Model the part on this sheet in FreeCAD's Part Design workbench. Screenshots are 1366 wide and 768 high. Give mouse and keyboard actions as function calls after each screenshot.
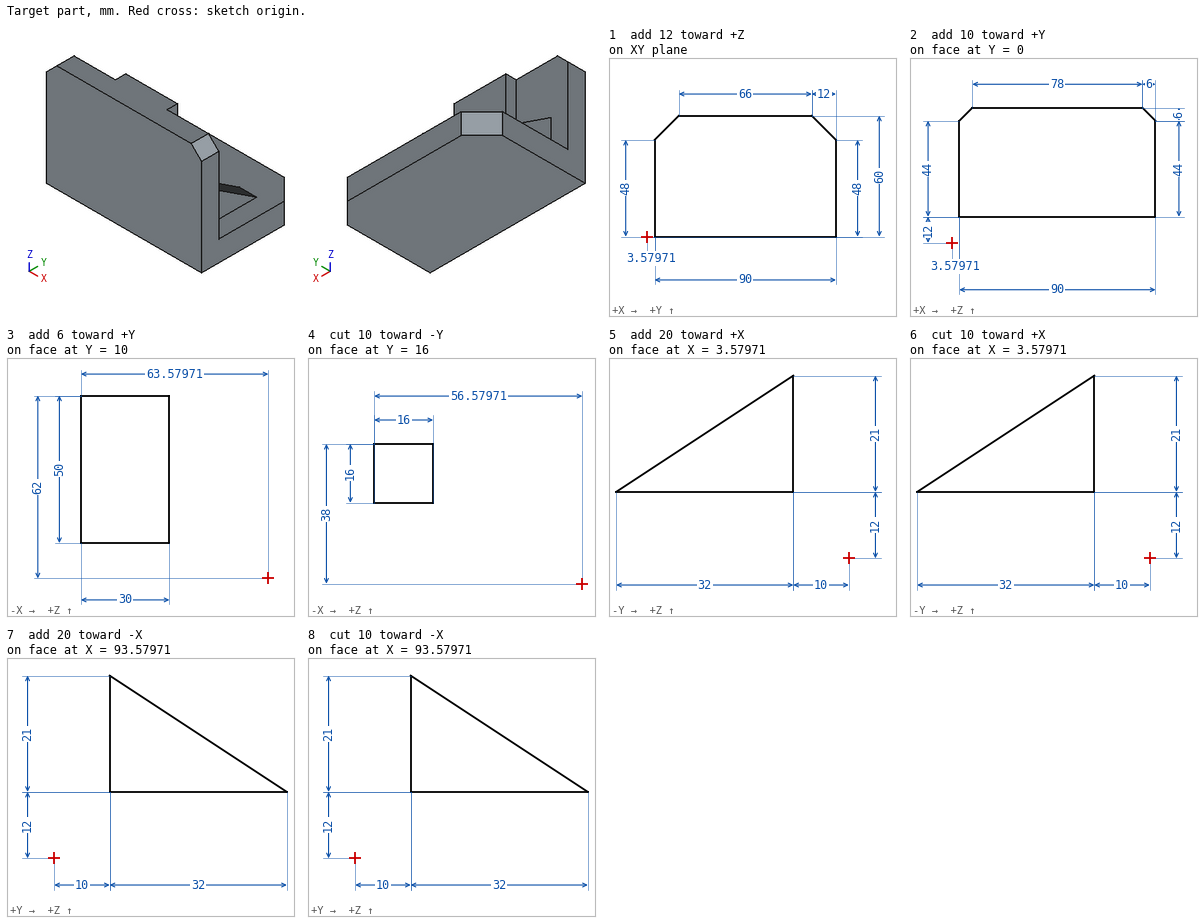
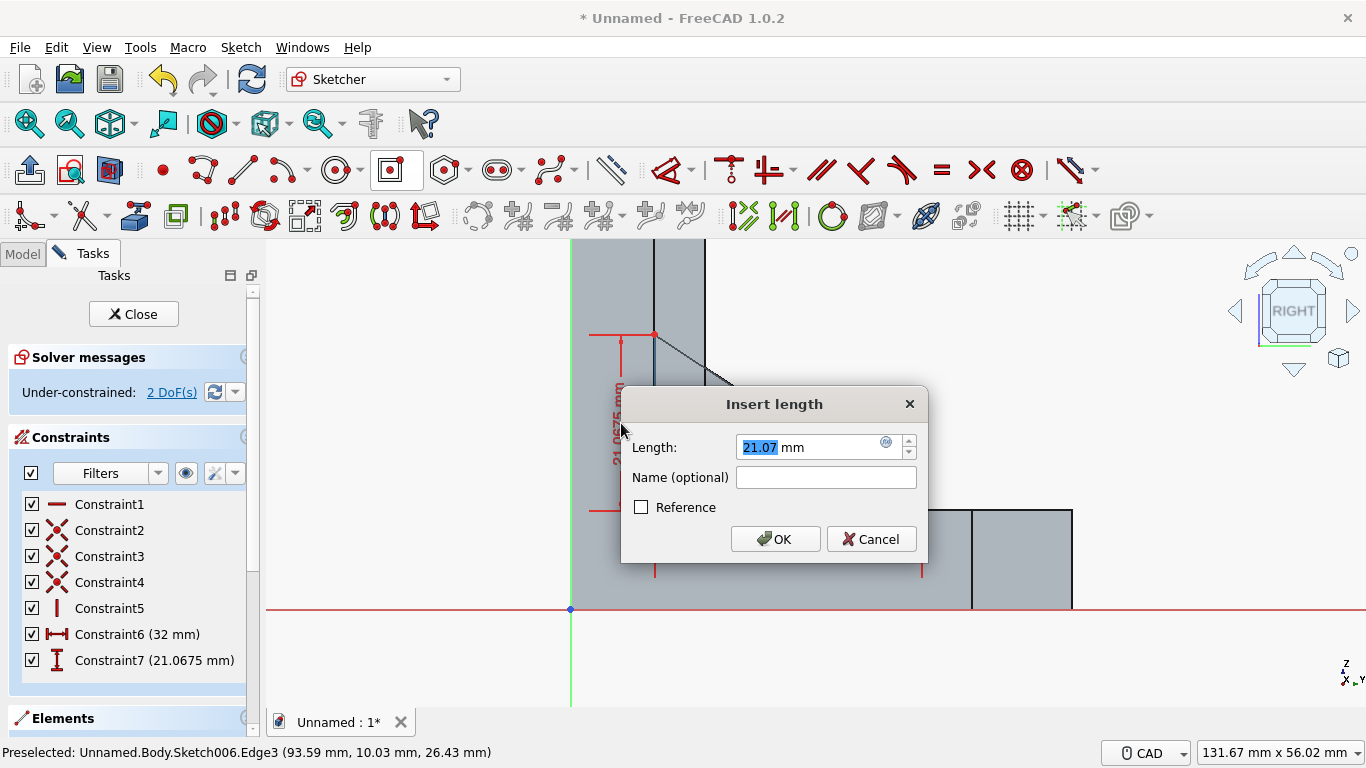
text(21)
key(Return)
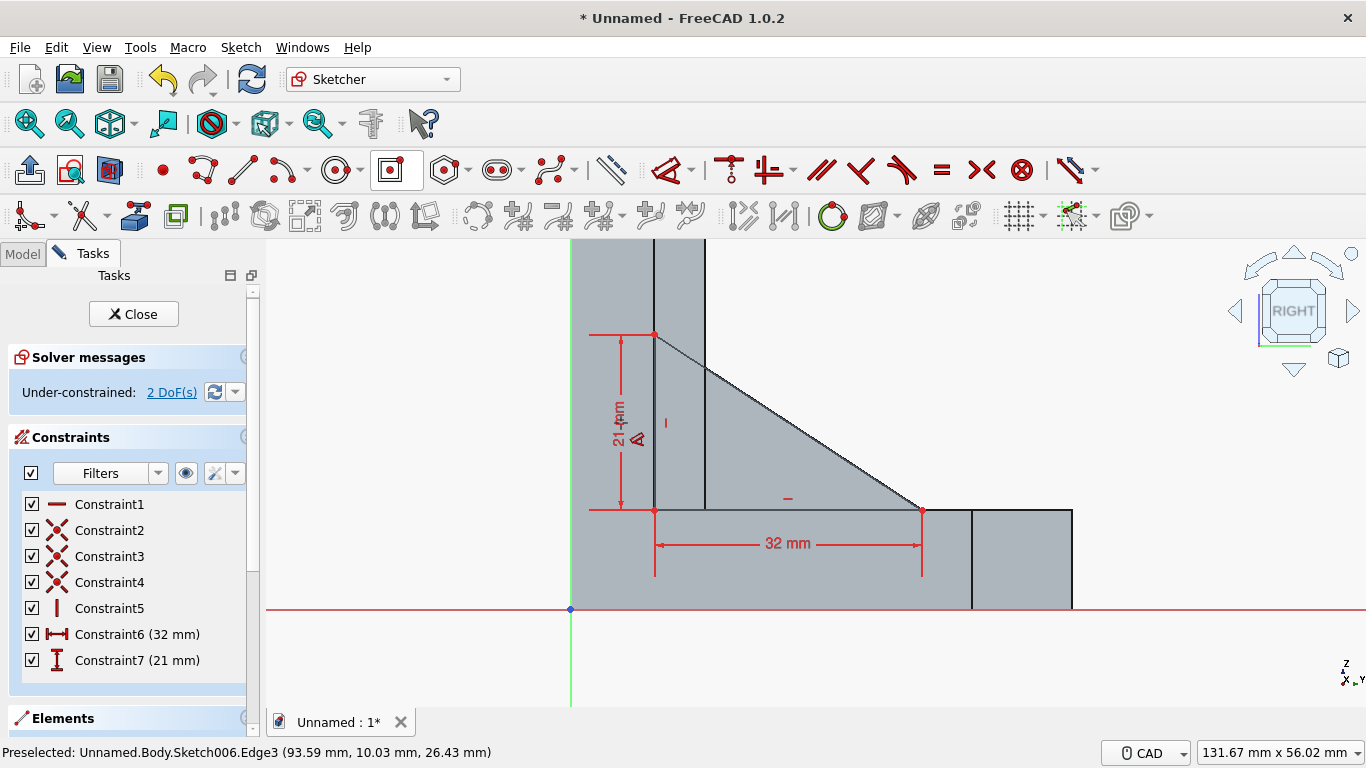
click(655, 510)
click(613, 644)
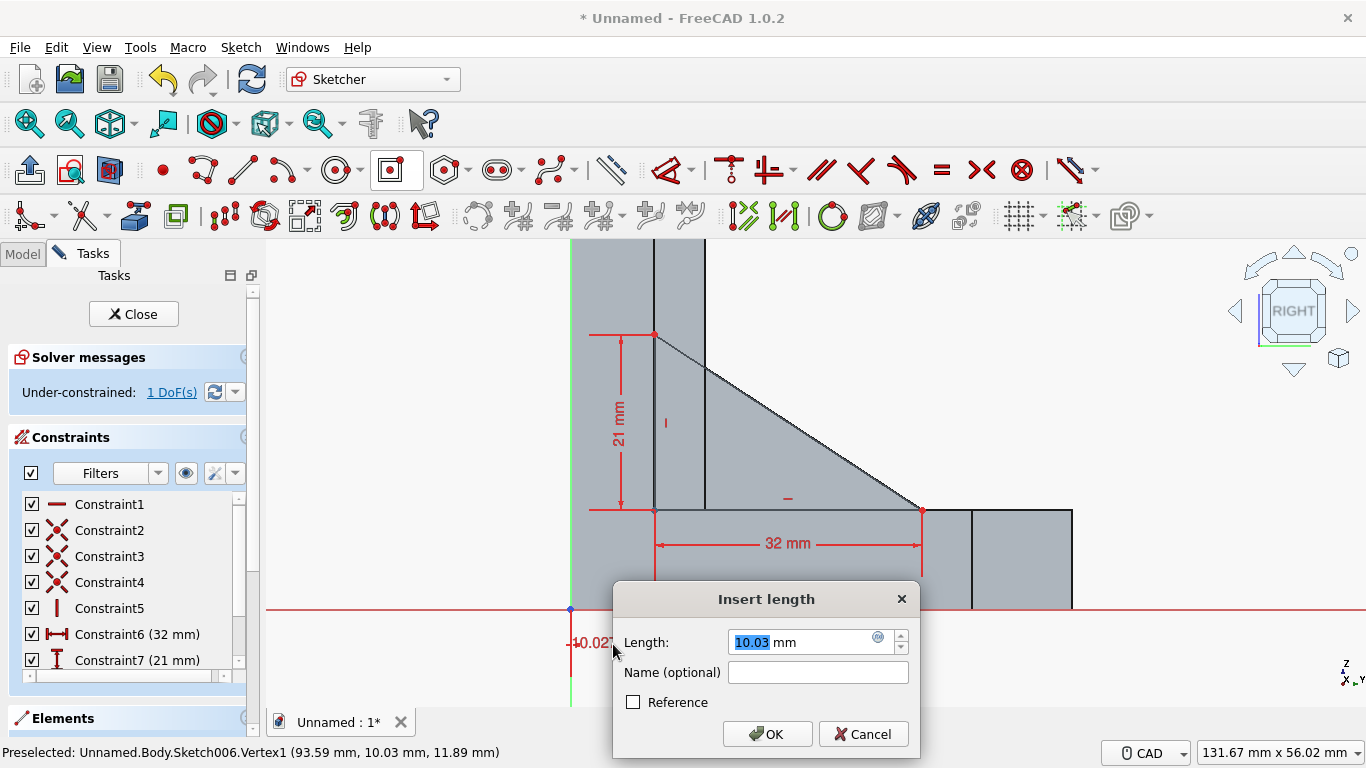
text(10)
key(Return)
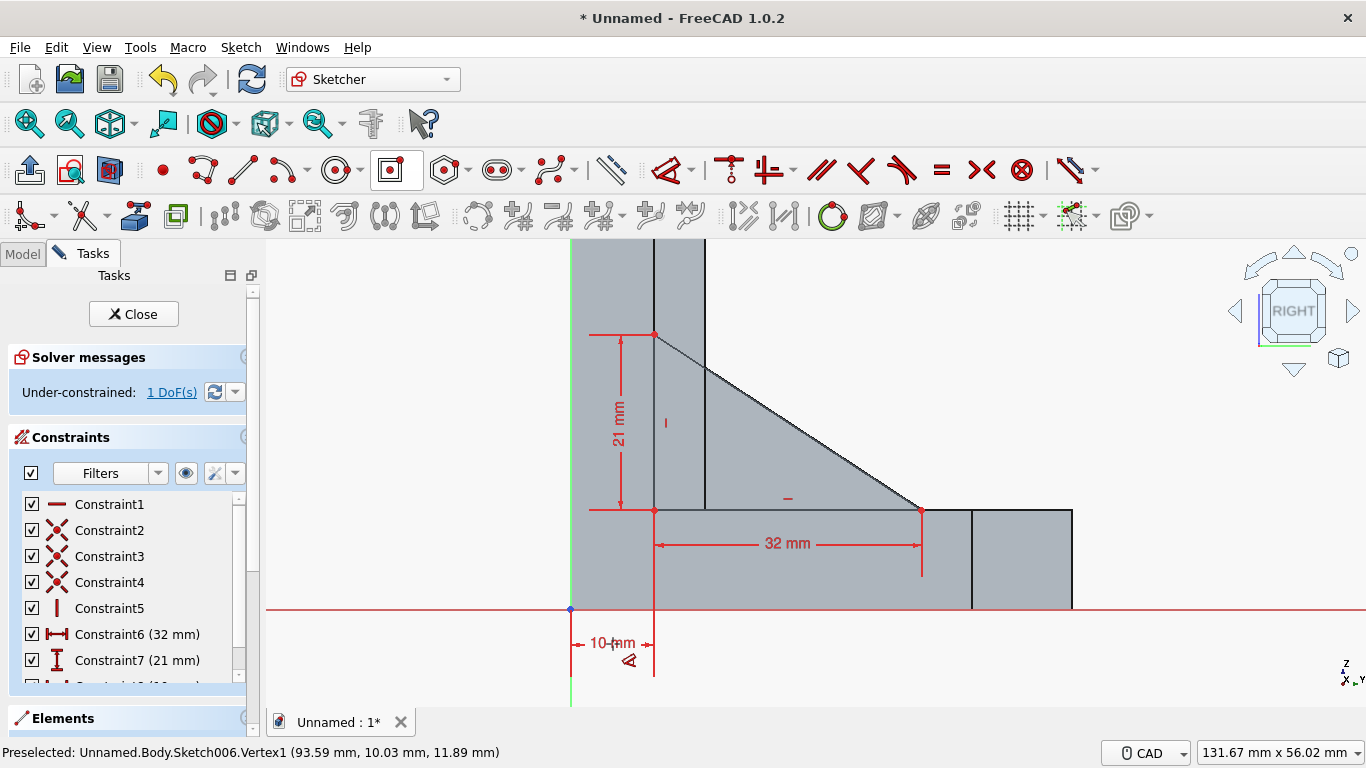
click(654, 510)
click(537, 560)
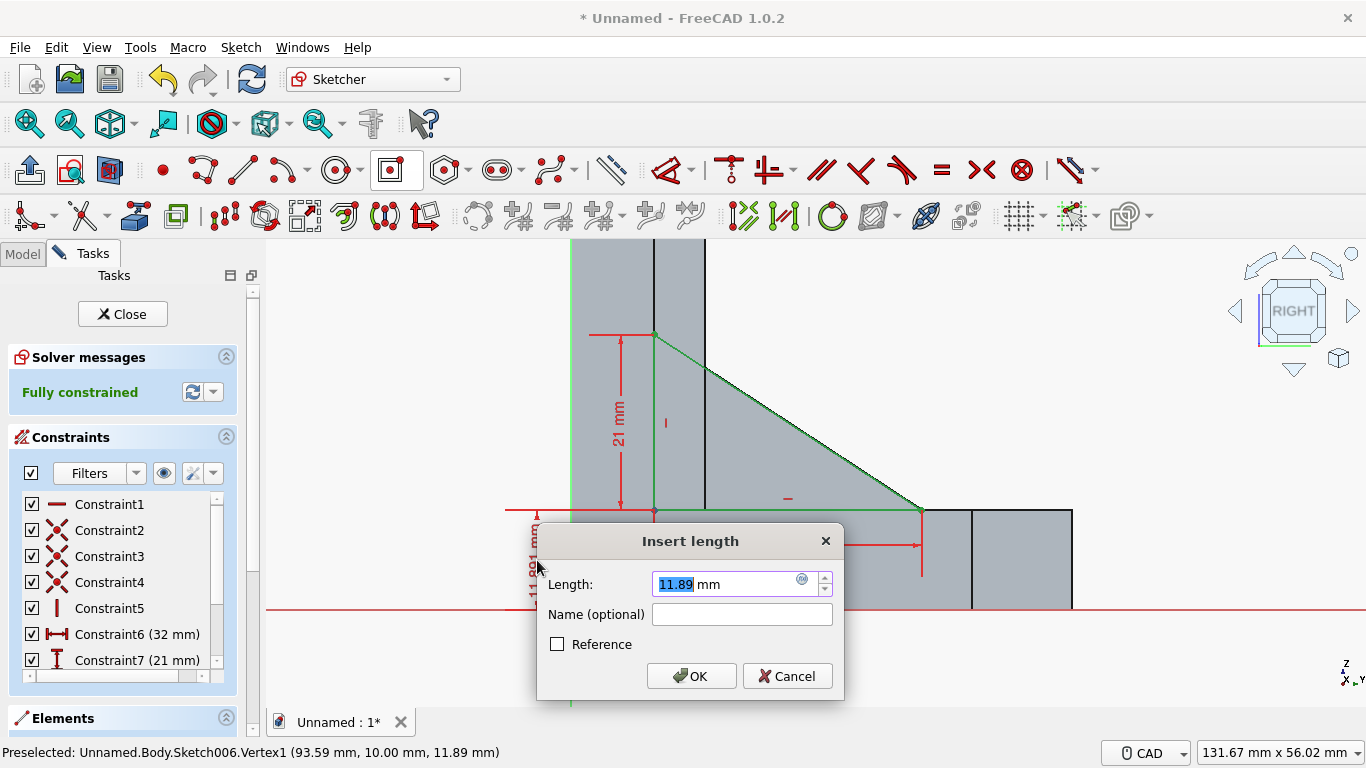
text(12)
key(Return)
key(Escape)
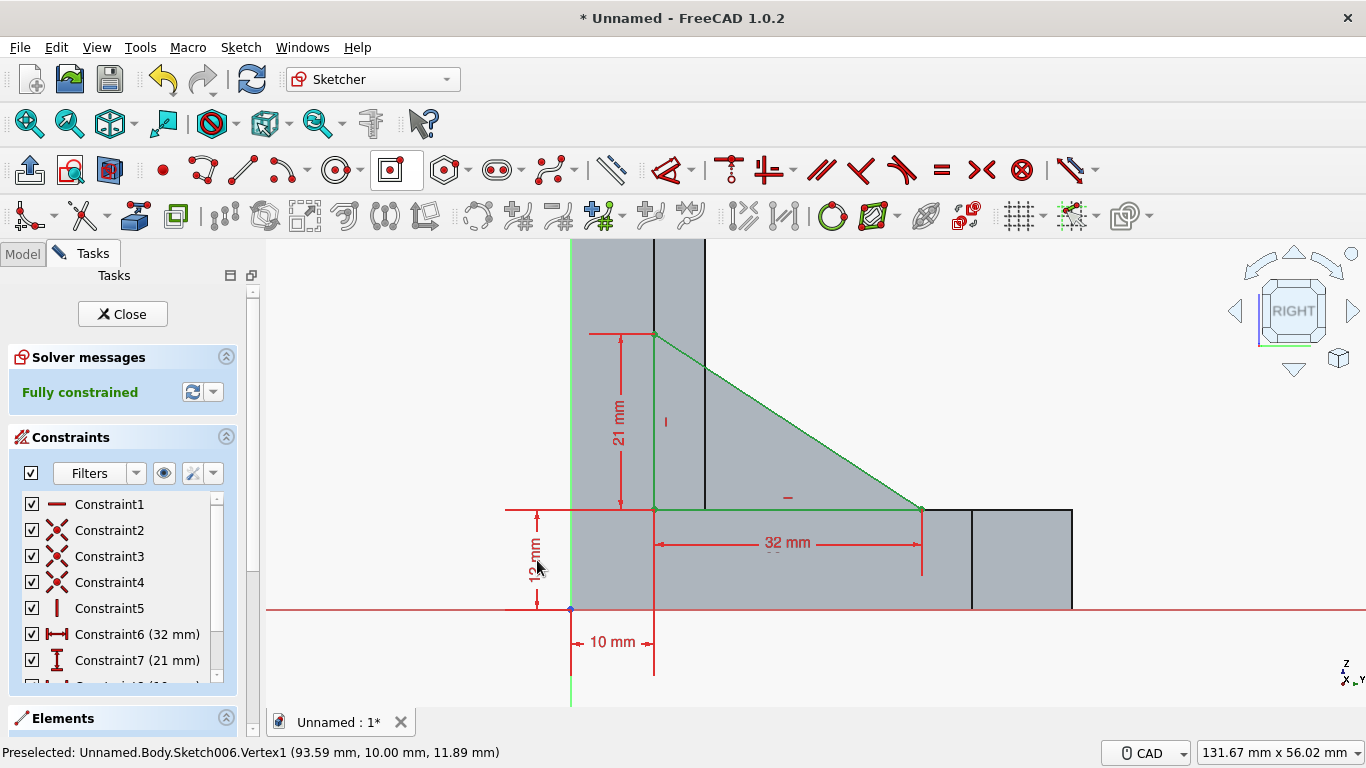
click(123, 314)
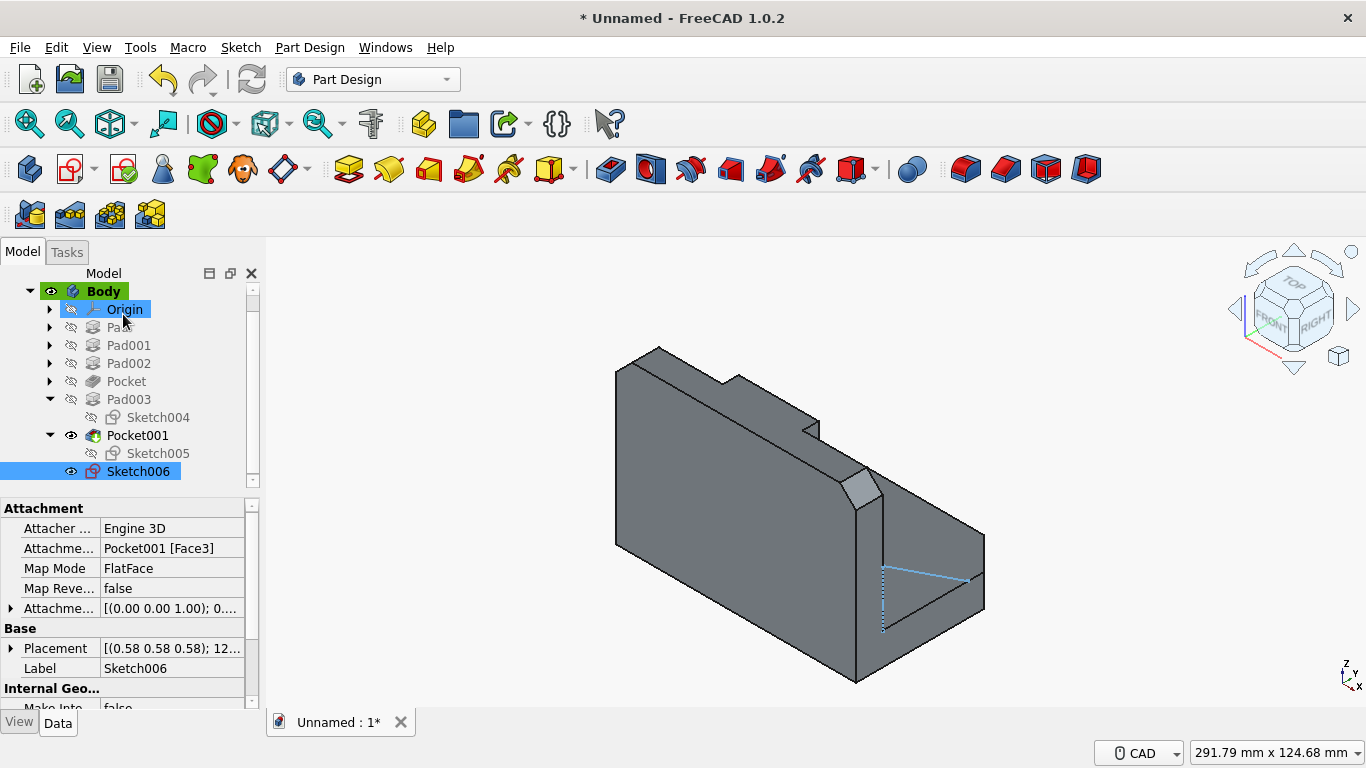
click(350, 170)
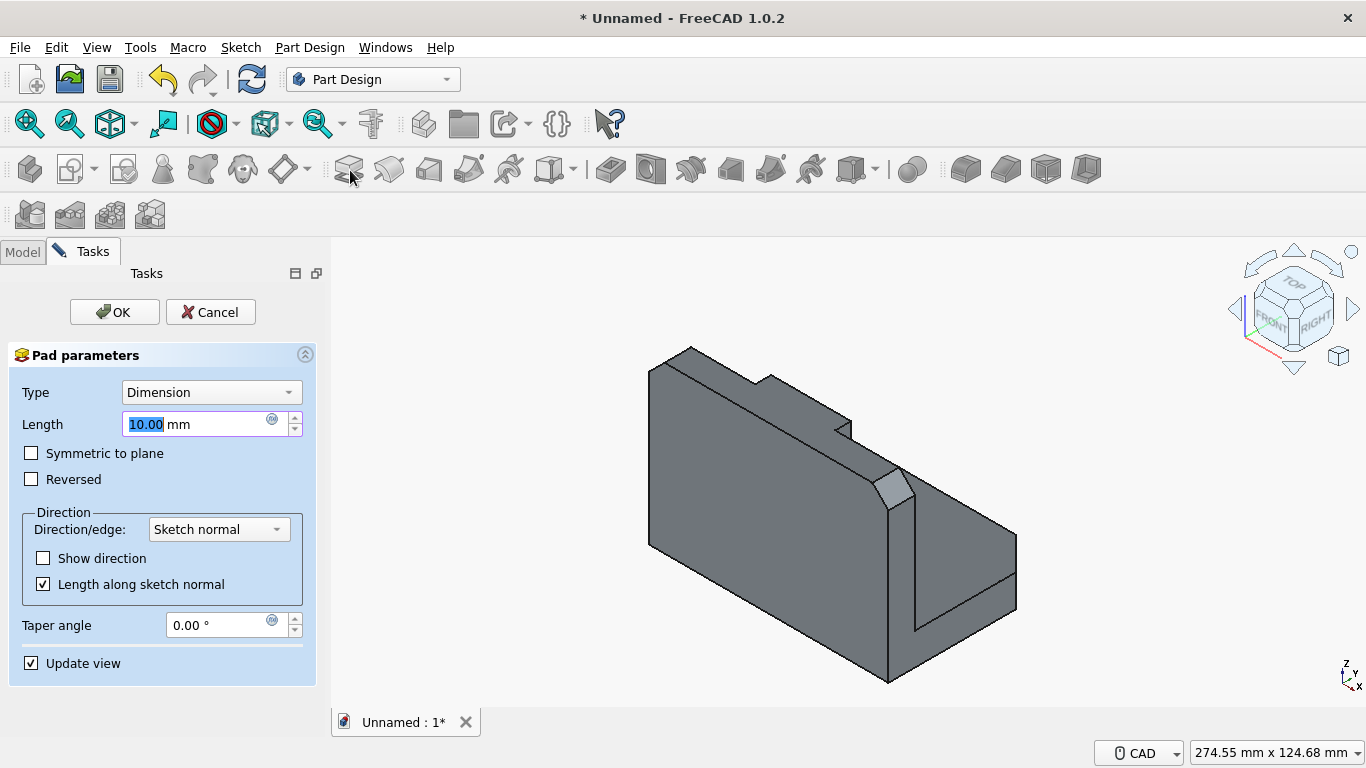
text(20)
key(Tab)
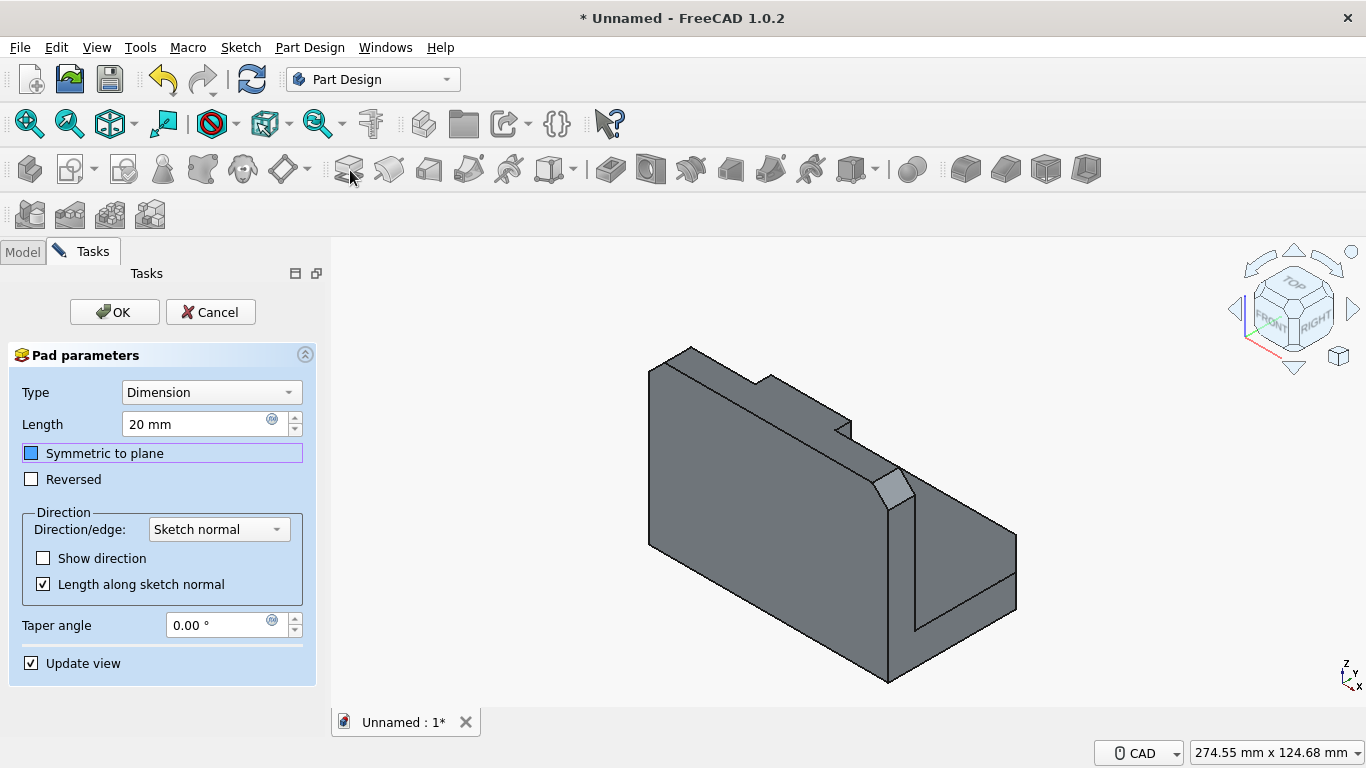
click(30, 479)